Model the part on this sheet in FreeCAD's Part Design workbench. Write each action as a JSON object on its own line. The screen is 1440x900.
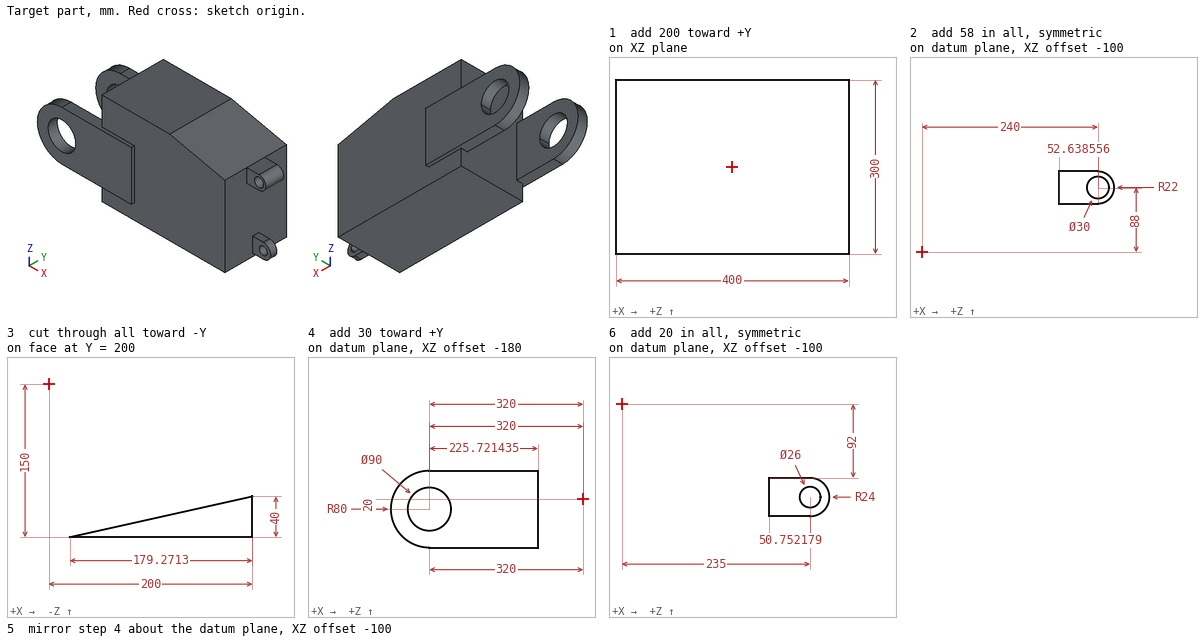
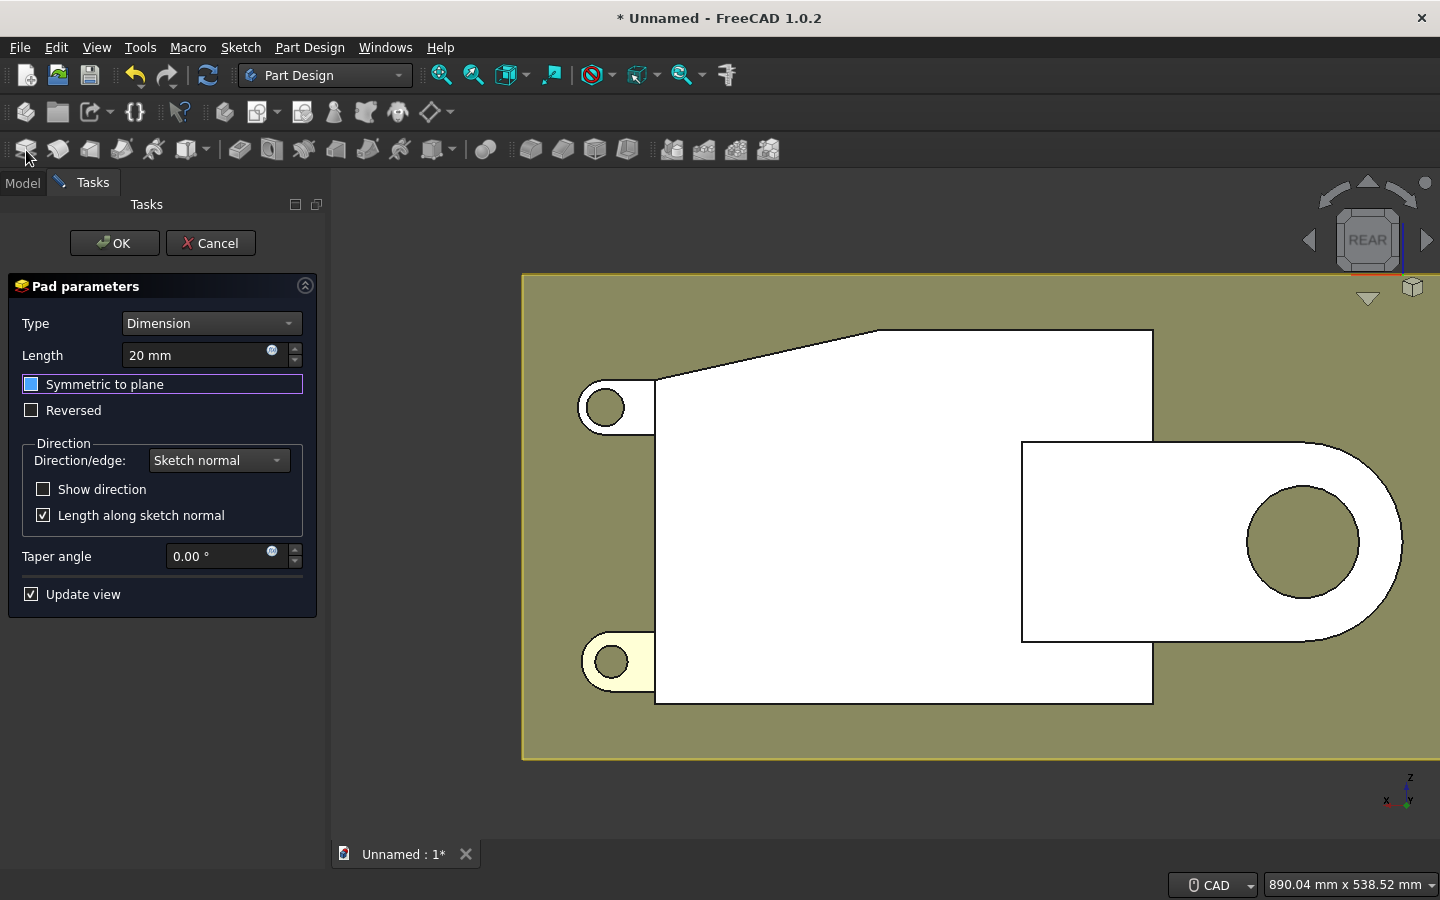
{"action": "left_click", "coordinate": [30, 384]}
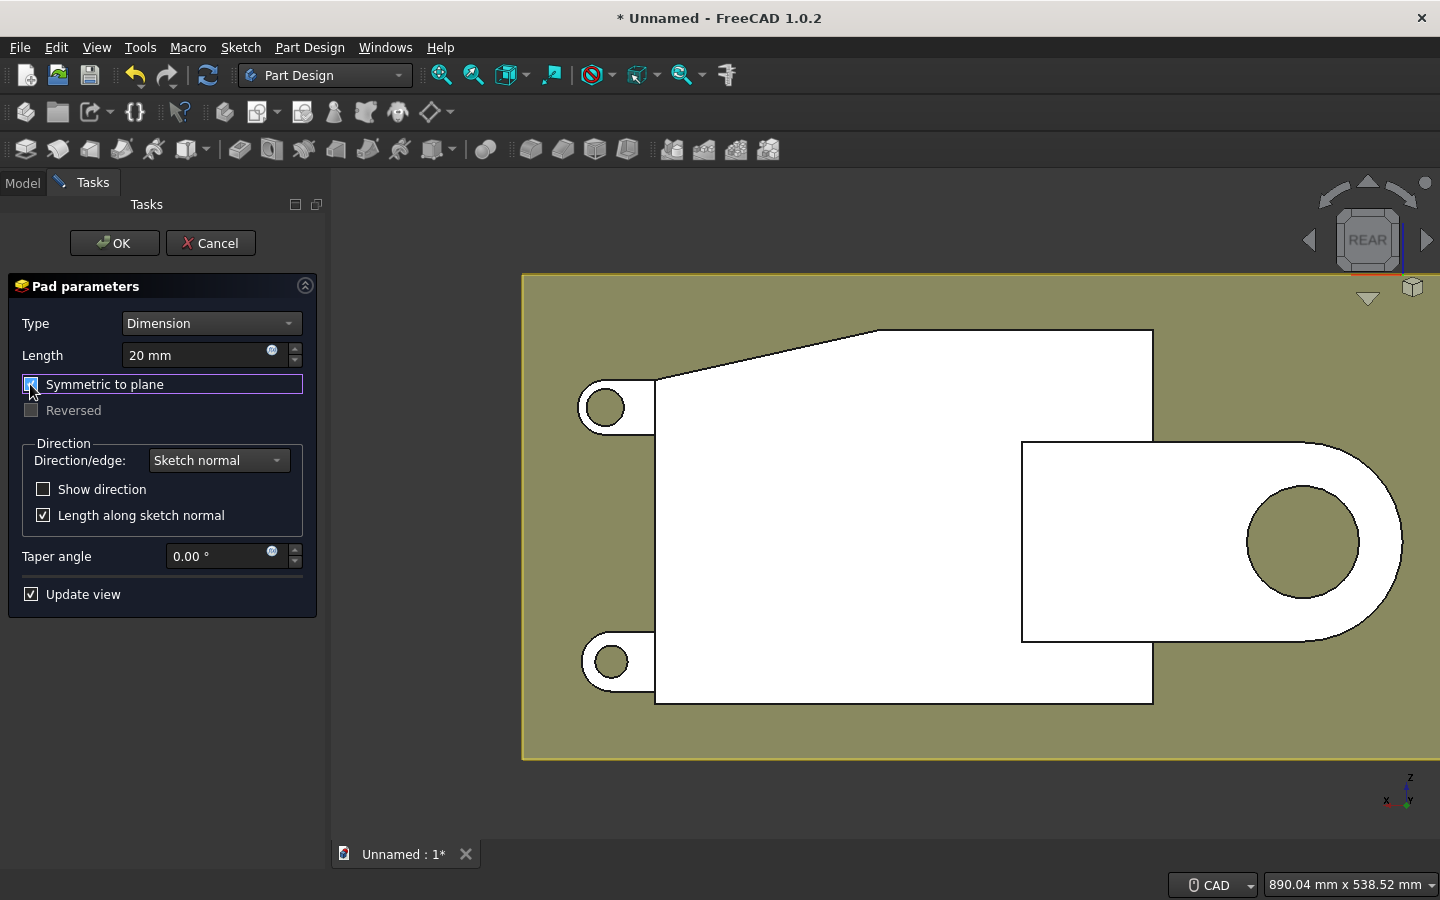
{"action": "left_click", "coordinate": [115, 243]}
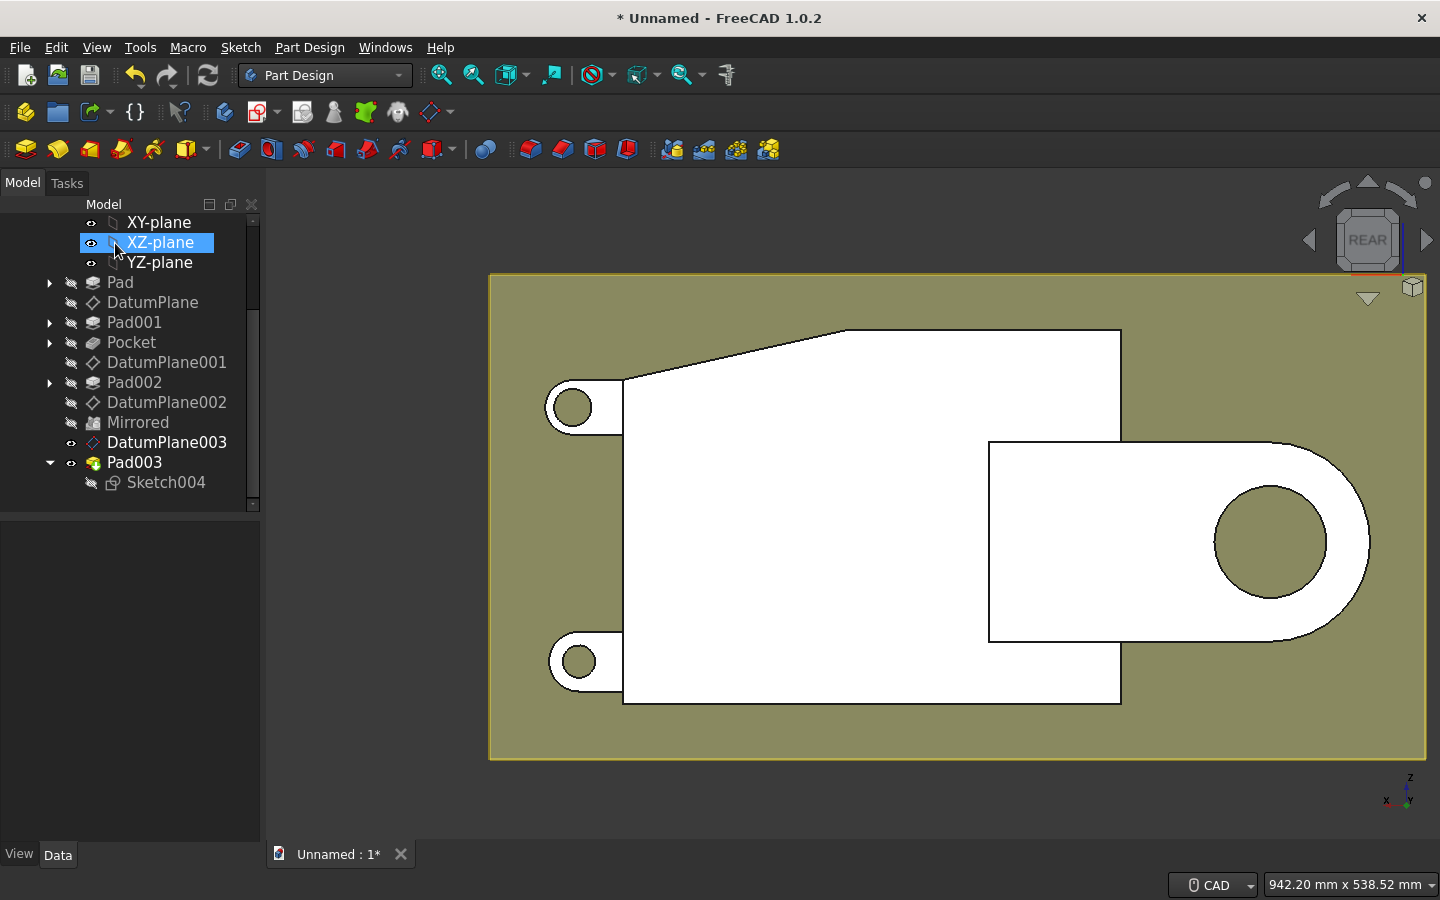
{"action": "left_click", "coordinate": [116, 443]}
{"action": "key", "text": "space"}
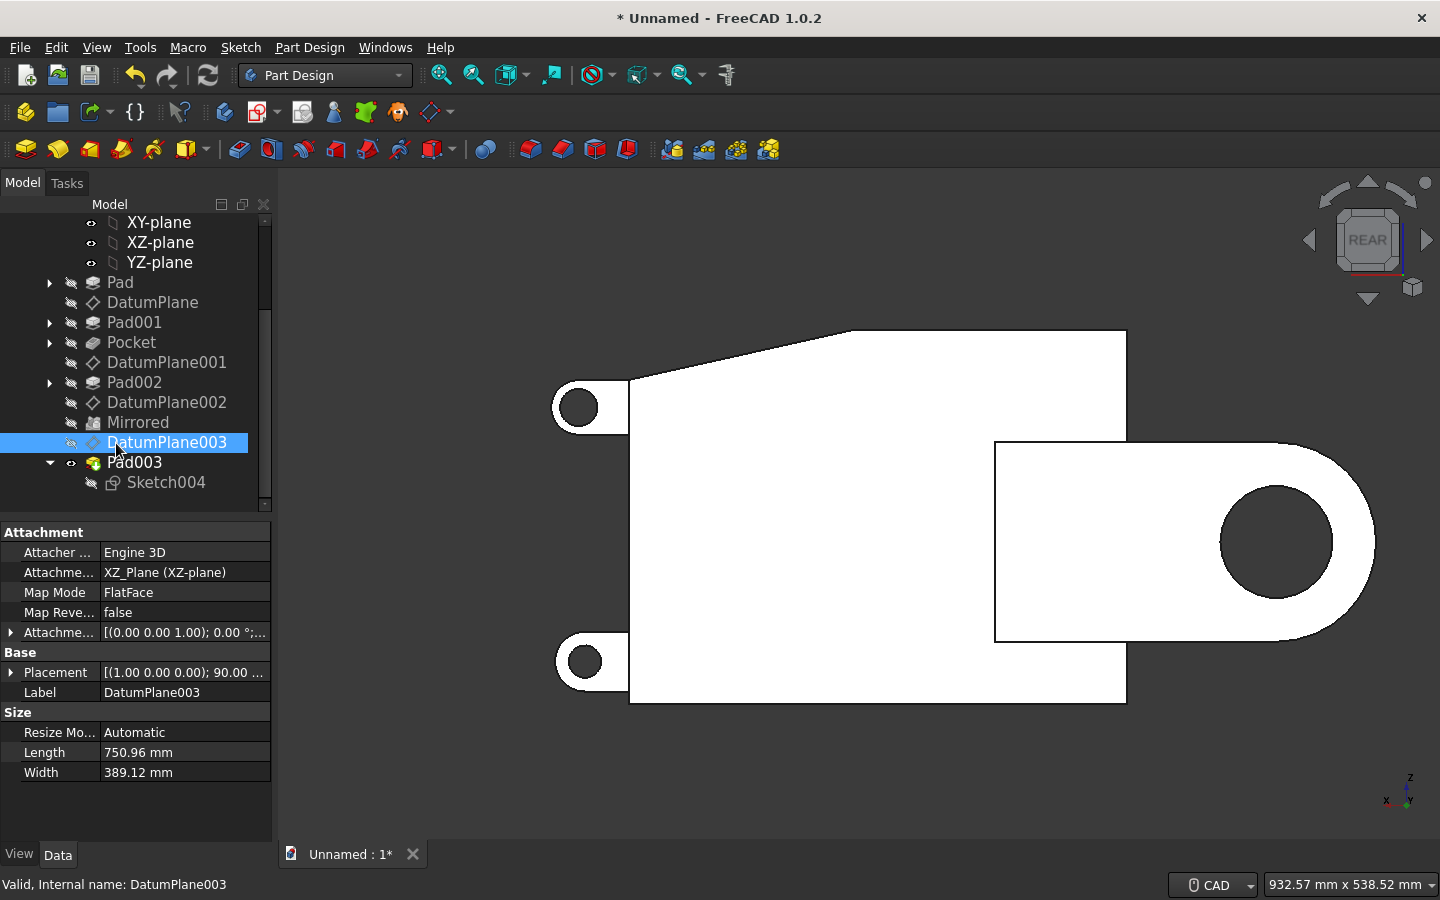
{"action": "key", "text": "0"}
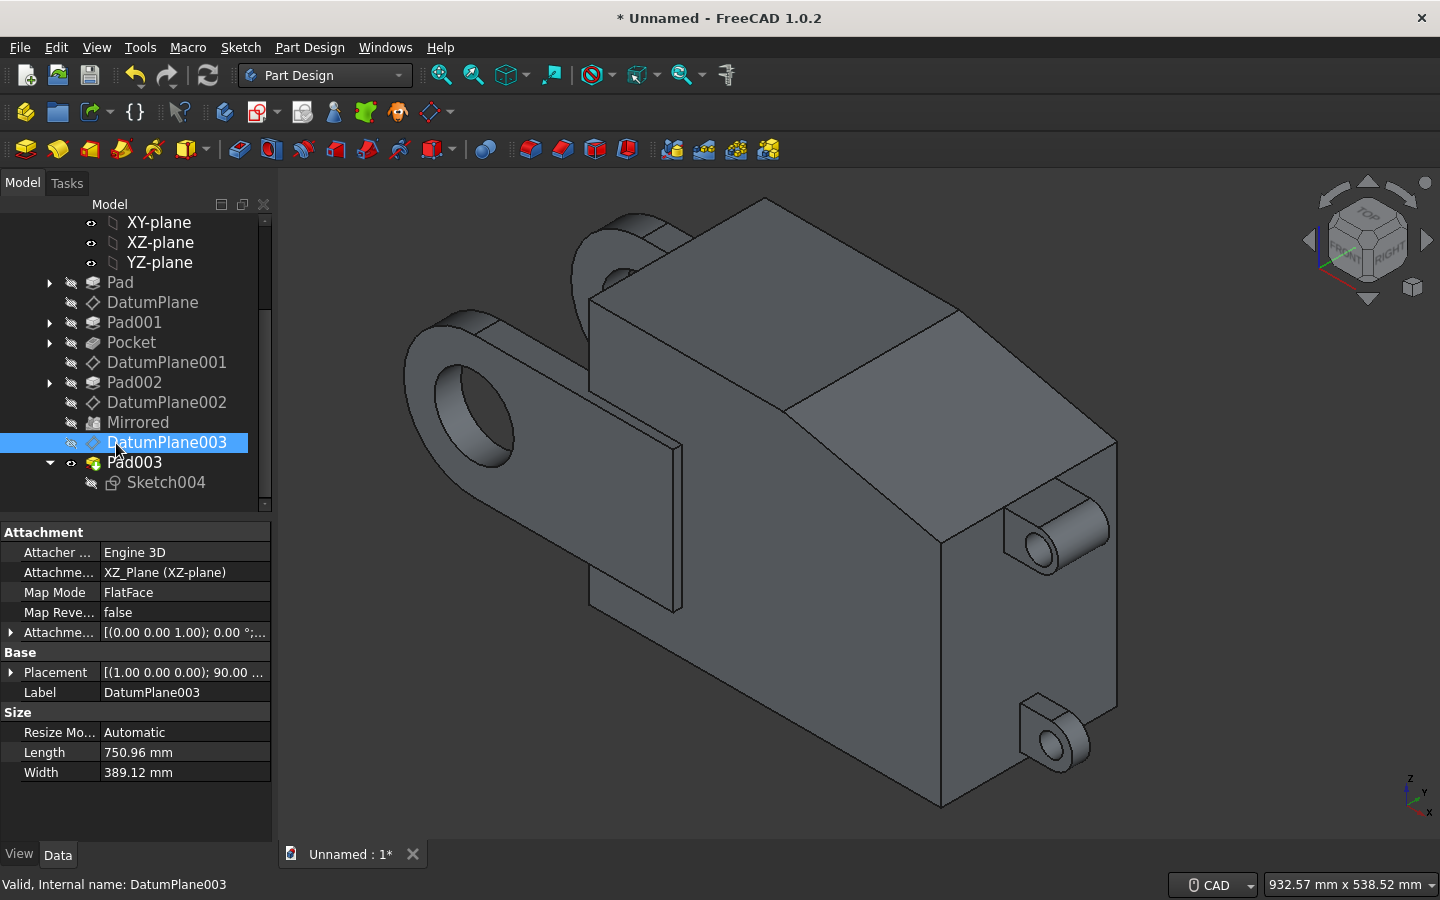
{"action": "left_click", "coordinate": [442, 76]}